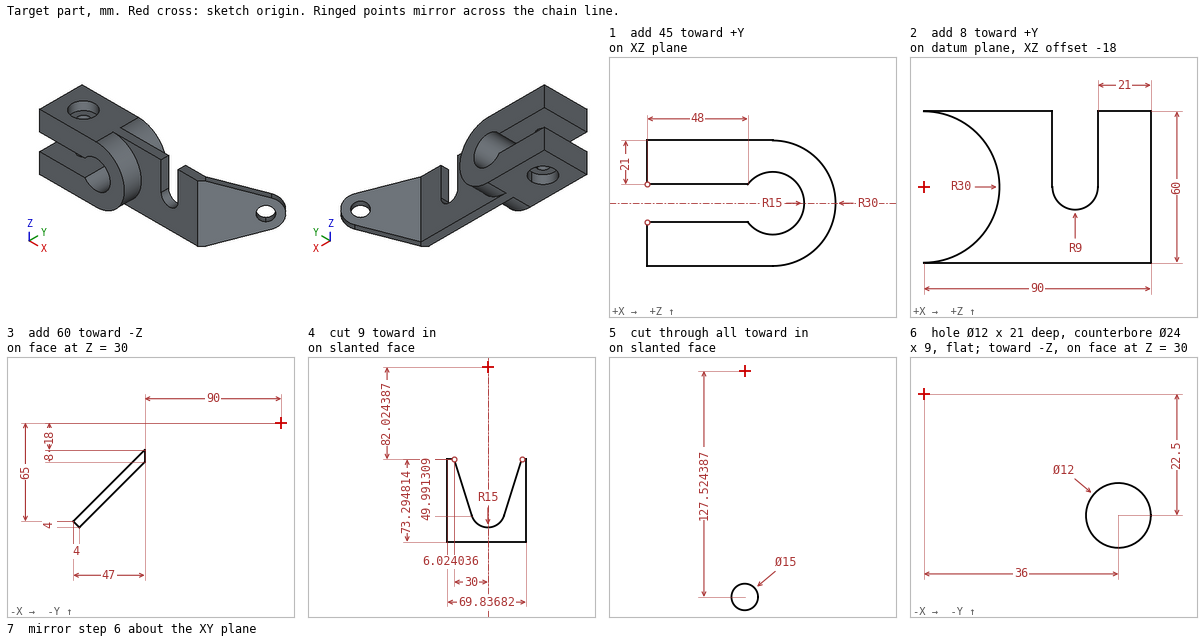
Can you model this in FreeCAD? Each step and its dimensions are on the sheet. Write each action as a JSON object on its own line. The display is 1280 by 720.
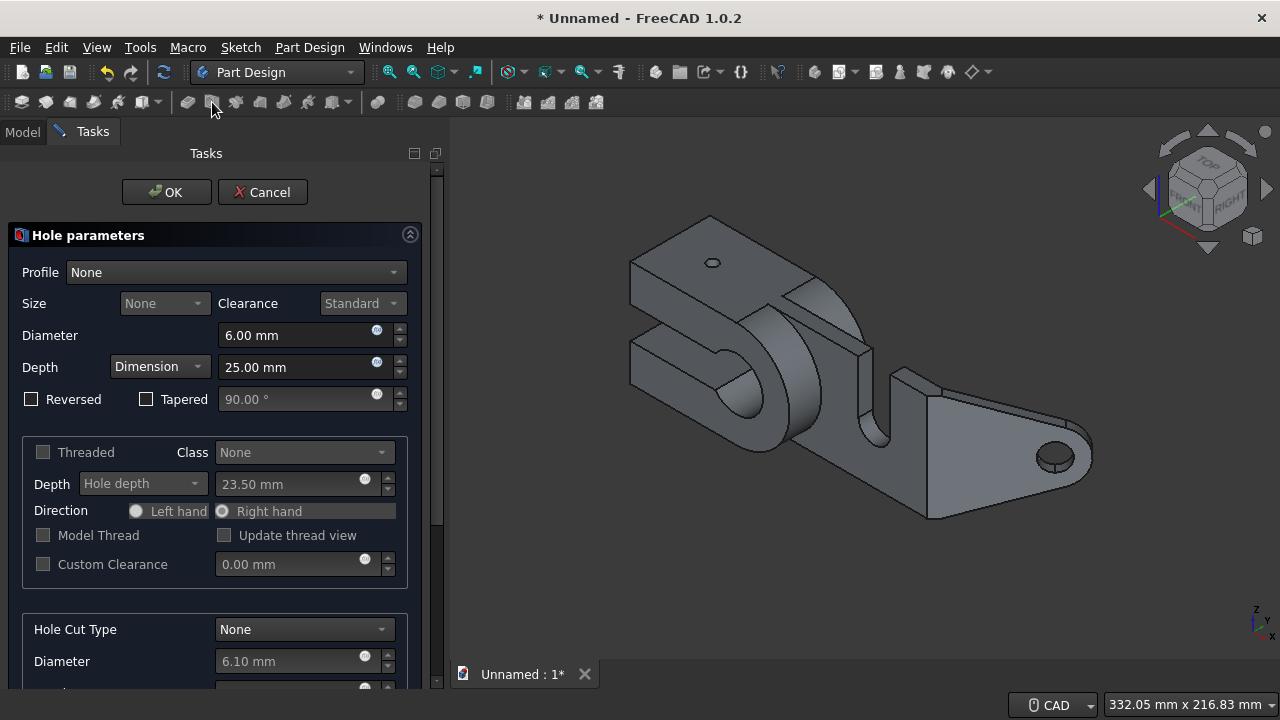
{"action": "triple_click", "coordinate": [305, 335]}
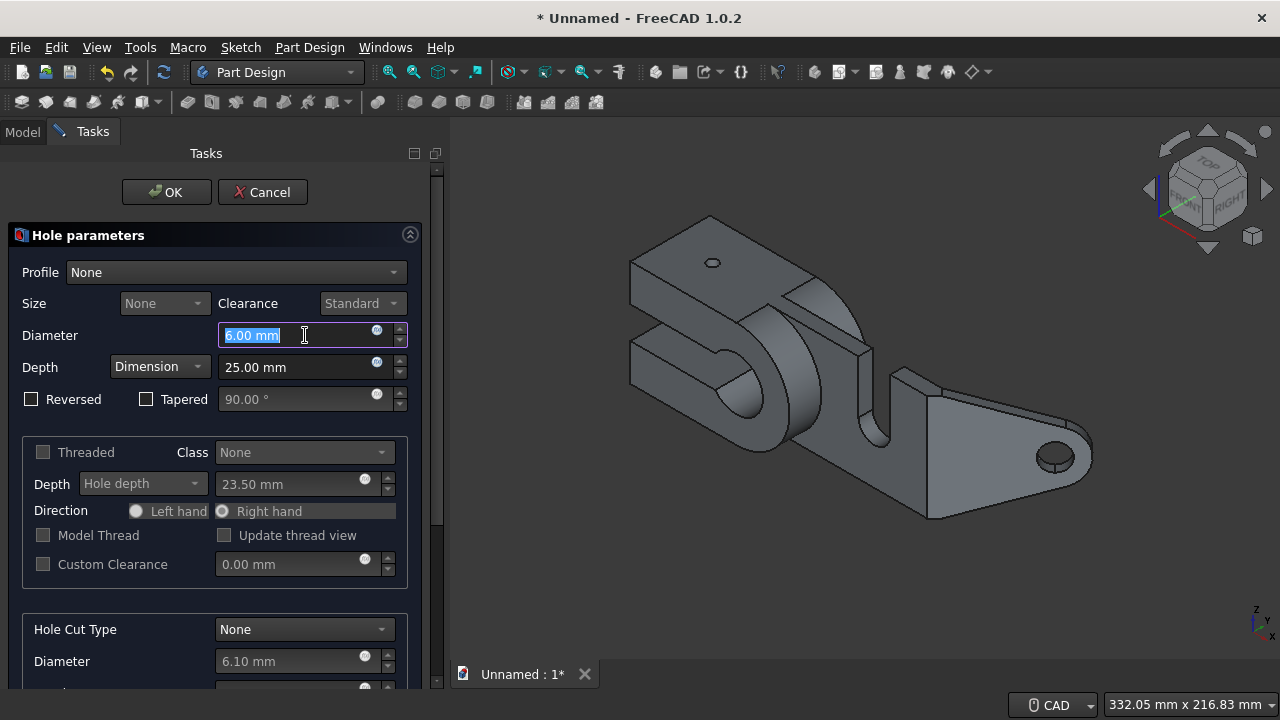
{"action": "type", "text": "12"}
{"action": "key", "text": "Tab"}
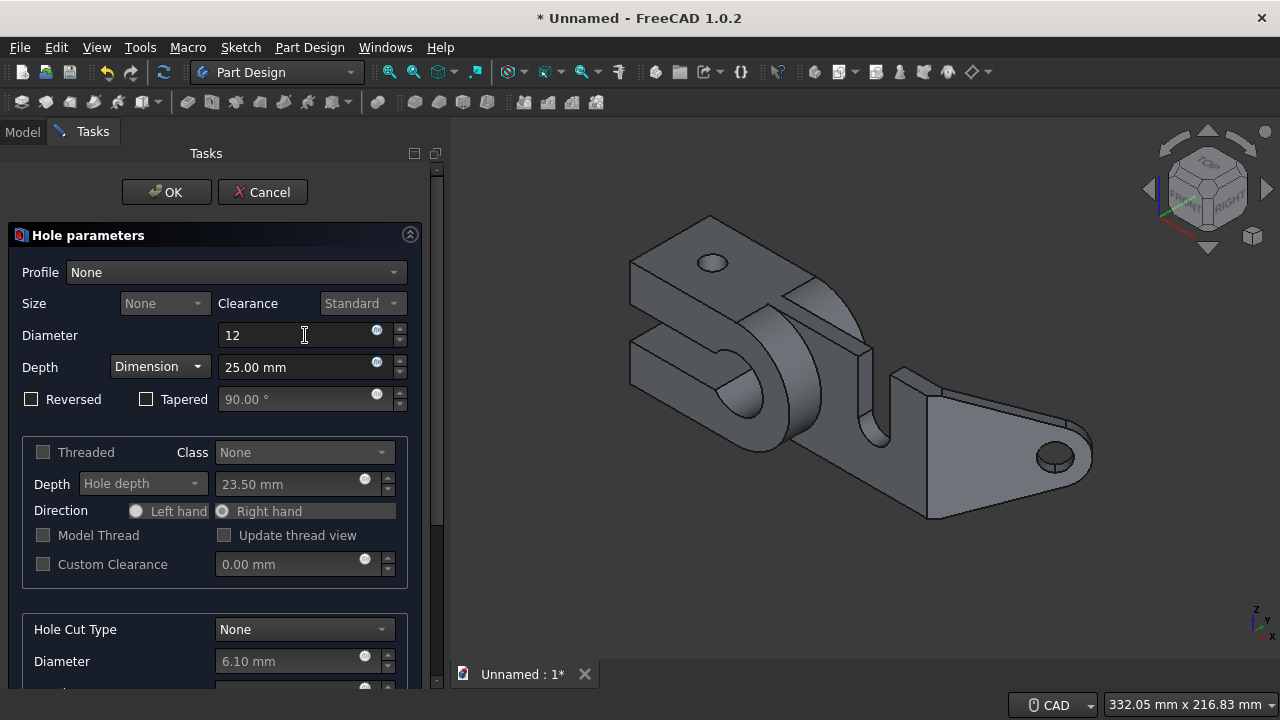
{"action": "triple_click", "coordinate": [305, 367]}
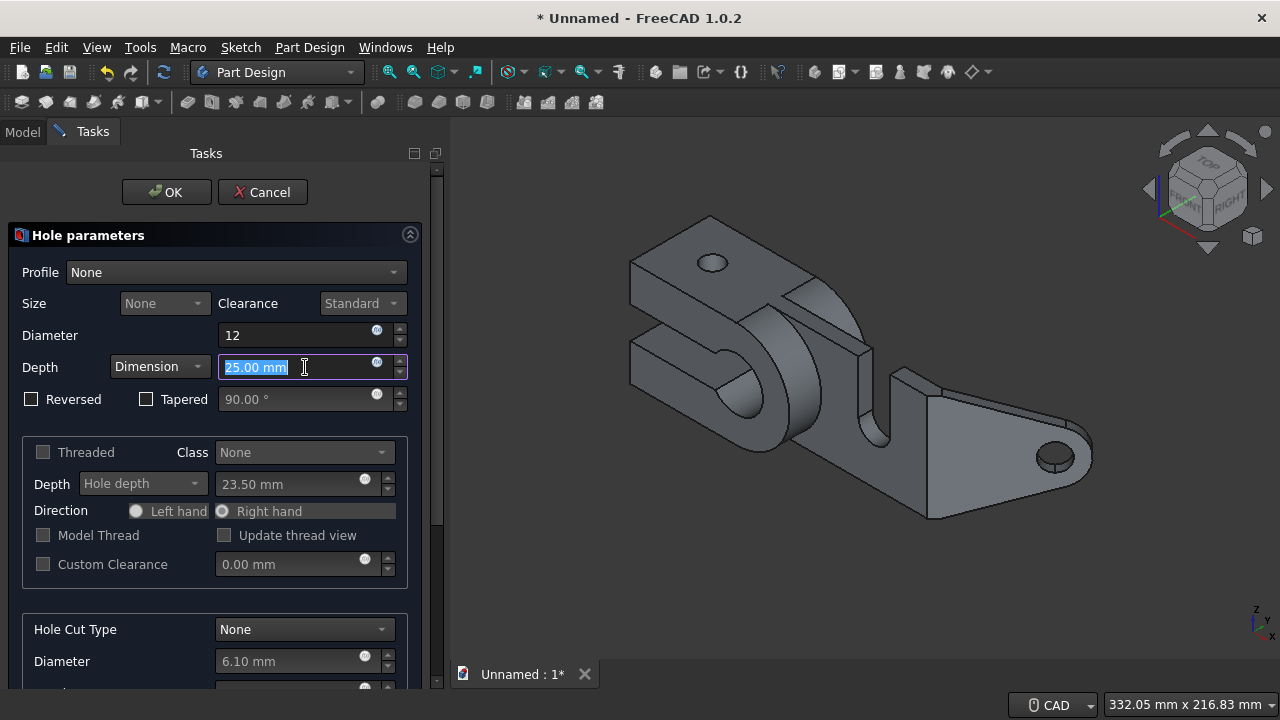
{"action": "type", "text": "21"}
{"action": "key", "text": "Tab"}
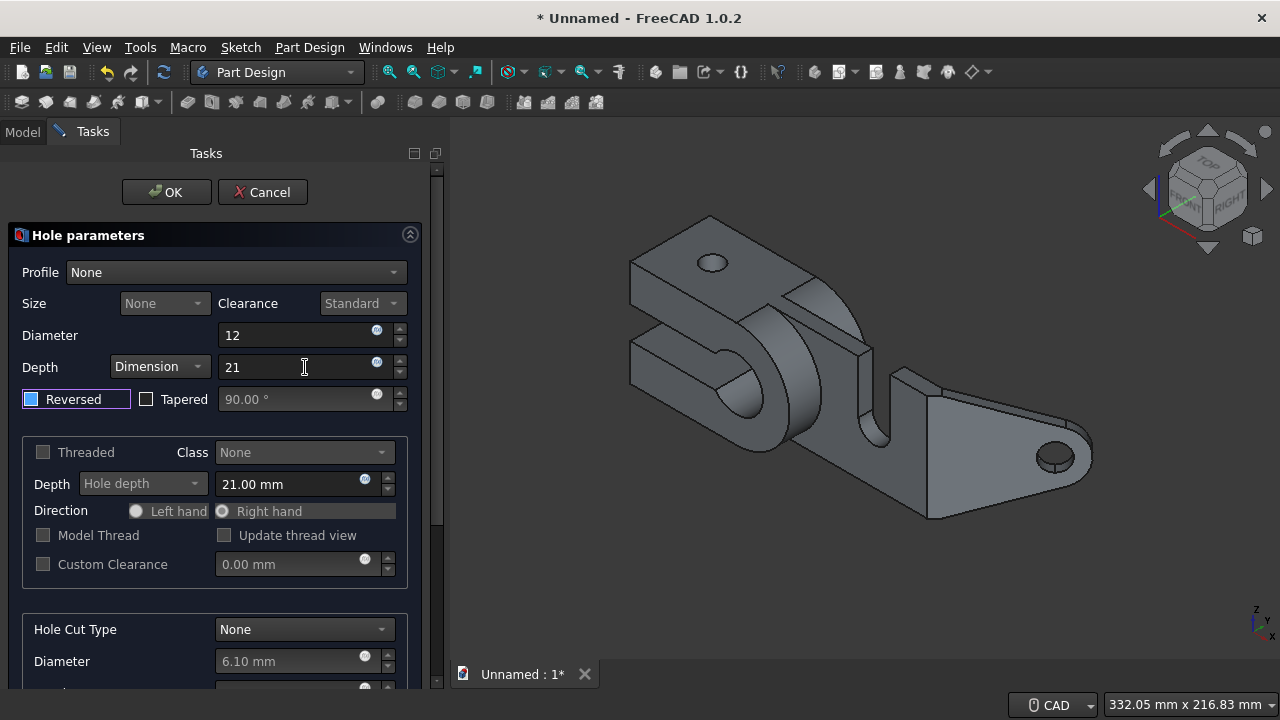
{"action": "left_click", "coordinate": [306, 630]}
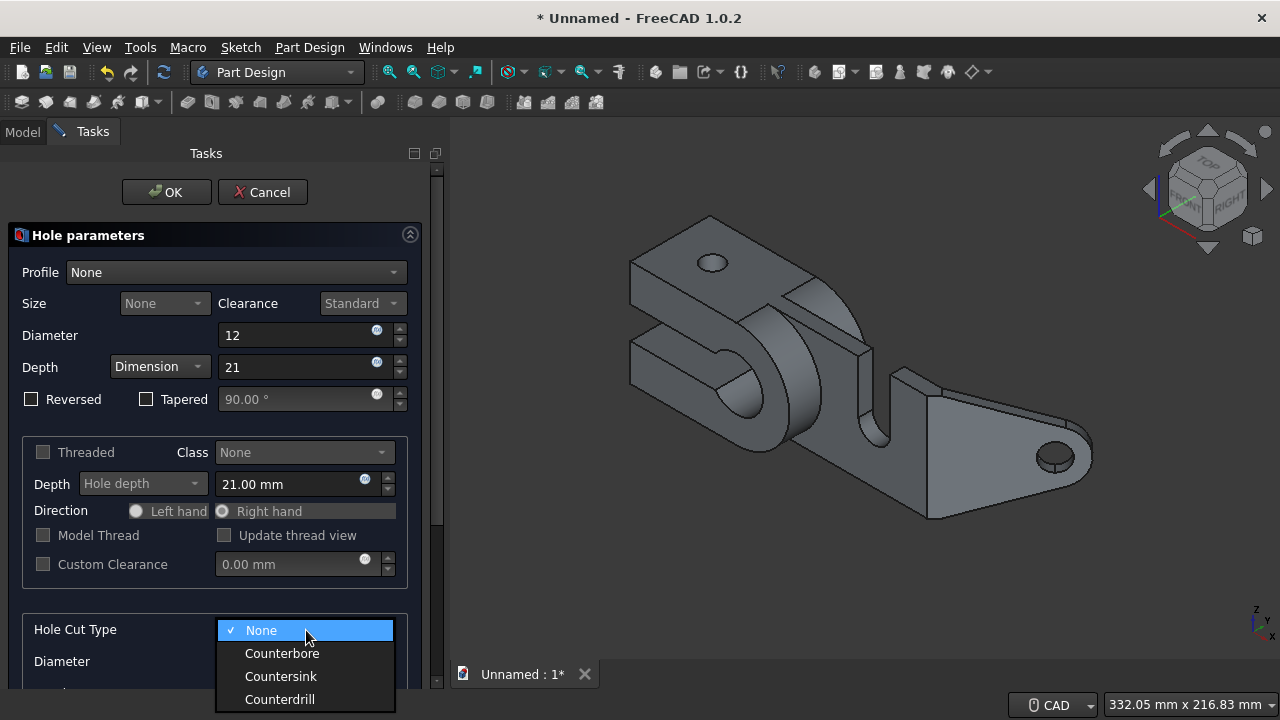
{"action": "left_click", "coordinate": [304, 654]}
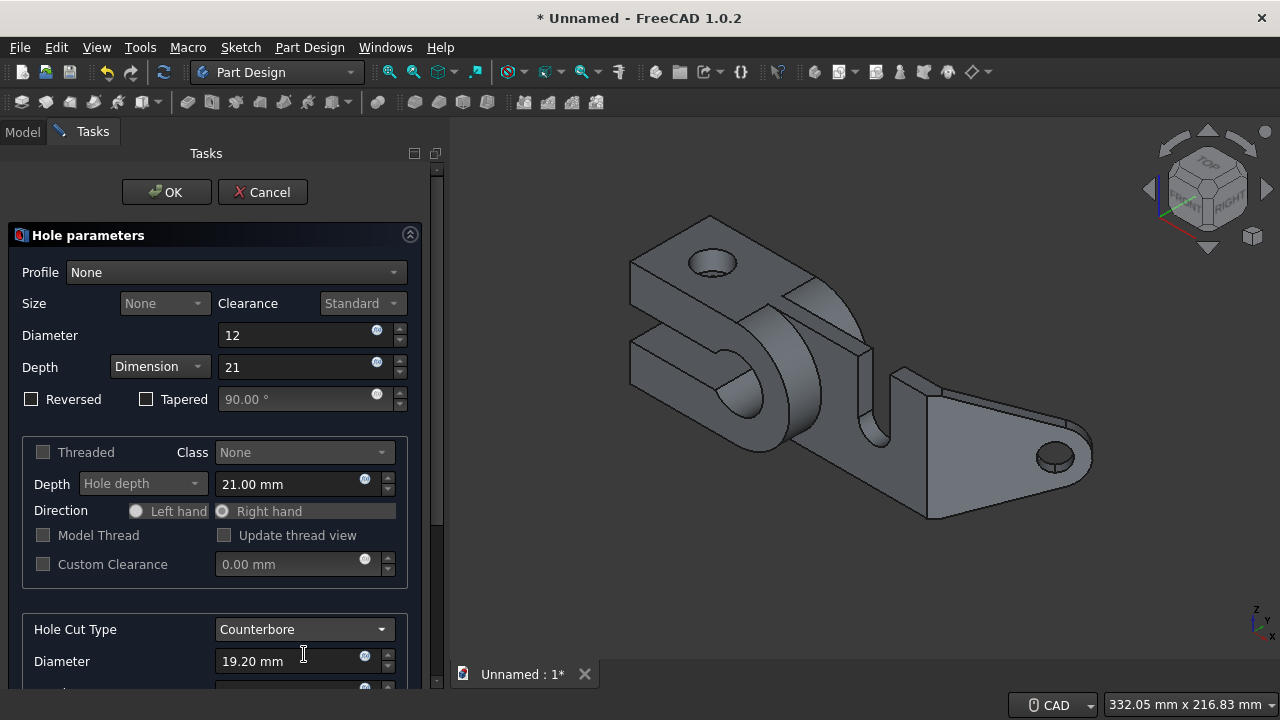
{"action": "triple_click", "coordinate": [298, 661]}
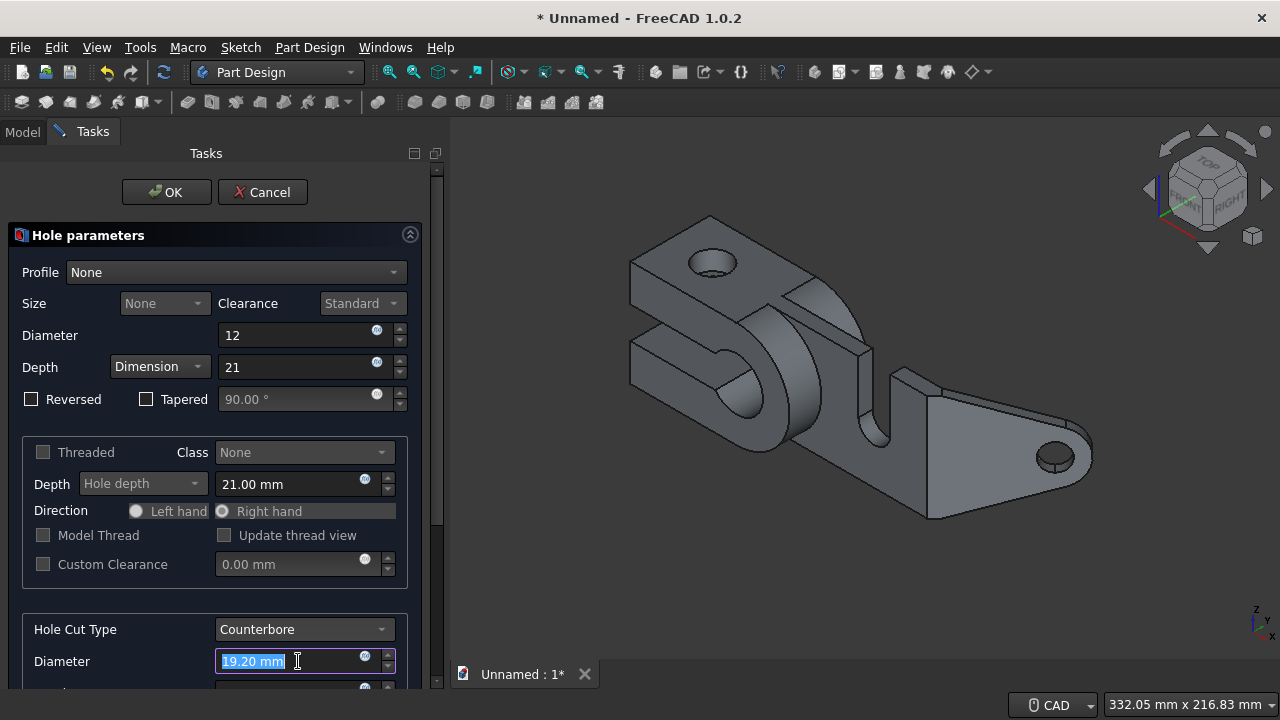
{"action": "type", "text": "24"}
{"action": "key", "text": "Tab"}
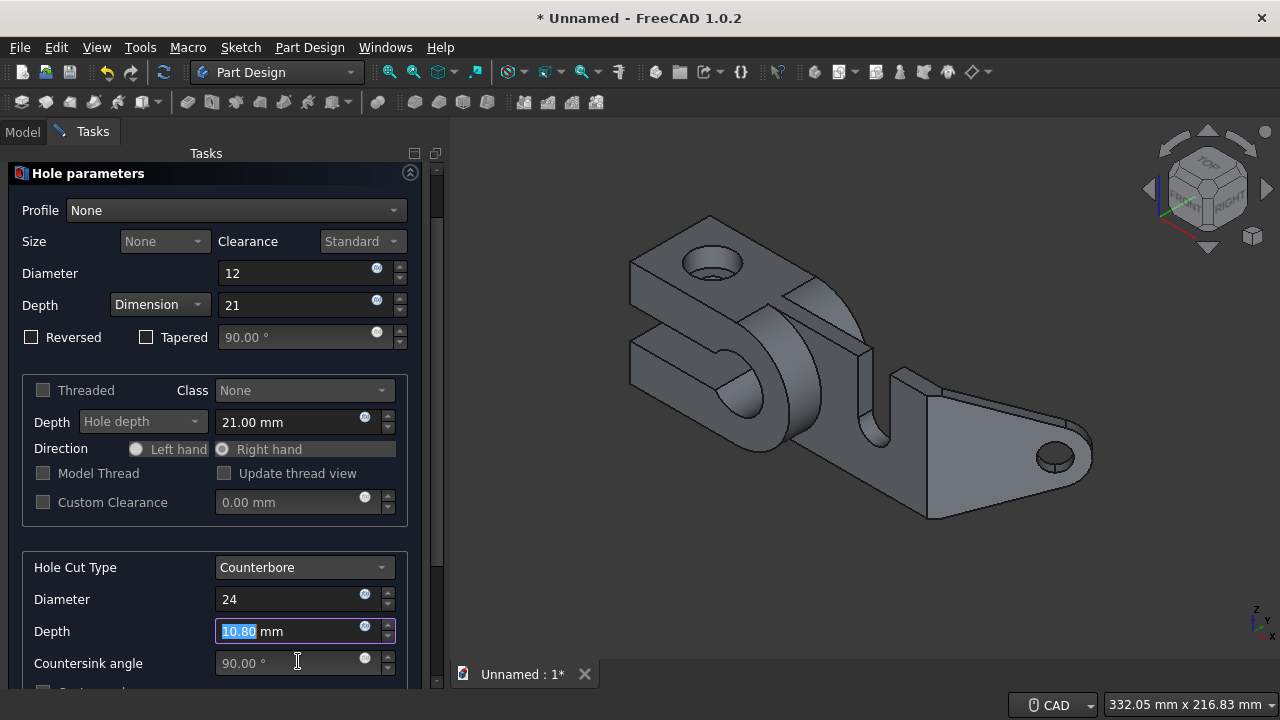
{"action": "type", "text": "9"}
{"action": "key", "text": "Tab"}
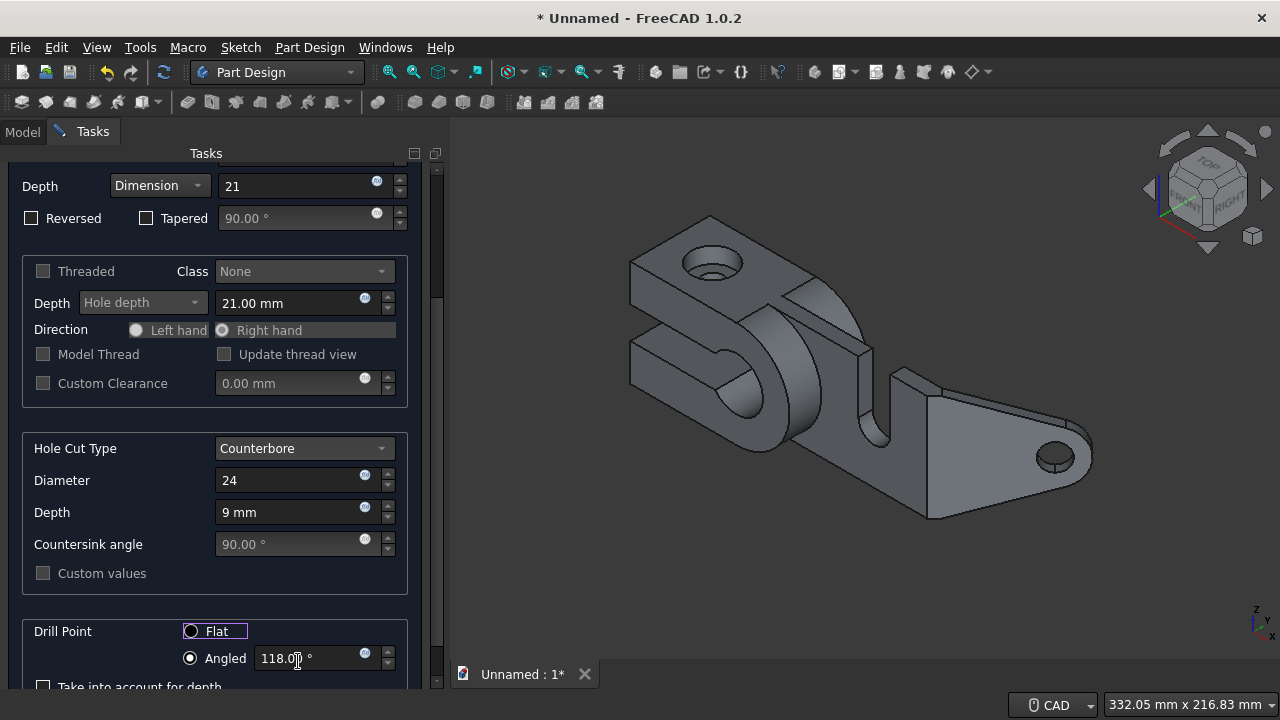
{"action": "left_click", "coordinate": [191, 631]}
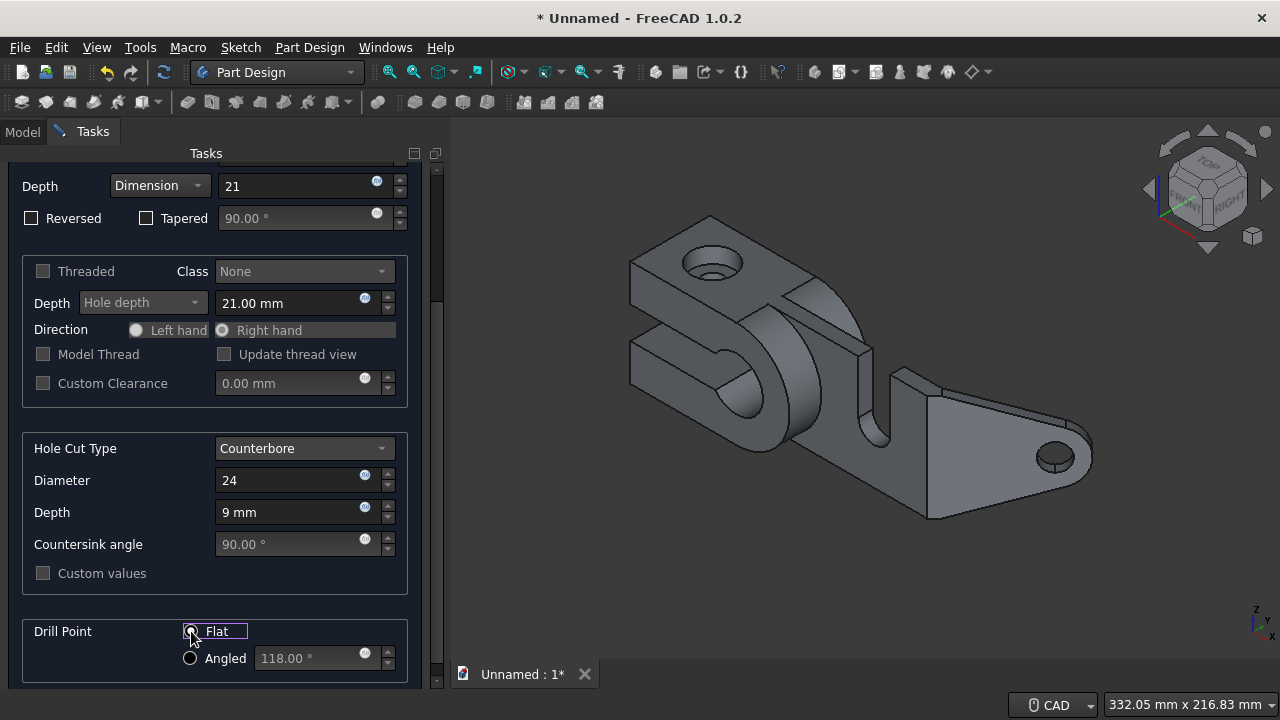
{"action": "scroll", "coordinate": [437, 426], "scroll_direction": "up", "scroll_amount": 4}